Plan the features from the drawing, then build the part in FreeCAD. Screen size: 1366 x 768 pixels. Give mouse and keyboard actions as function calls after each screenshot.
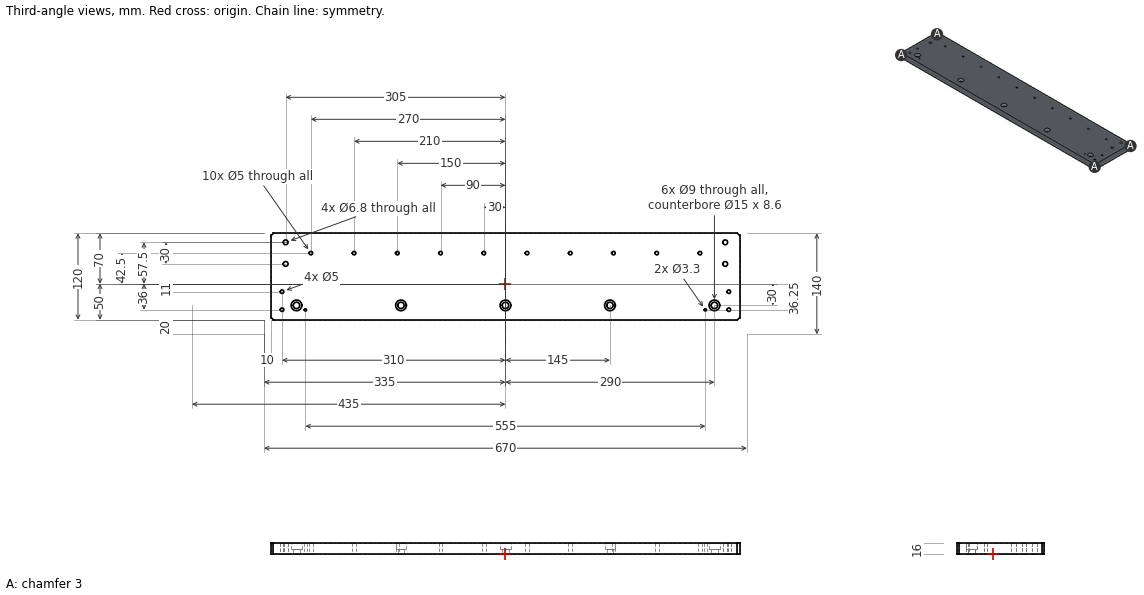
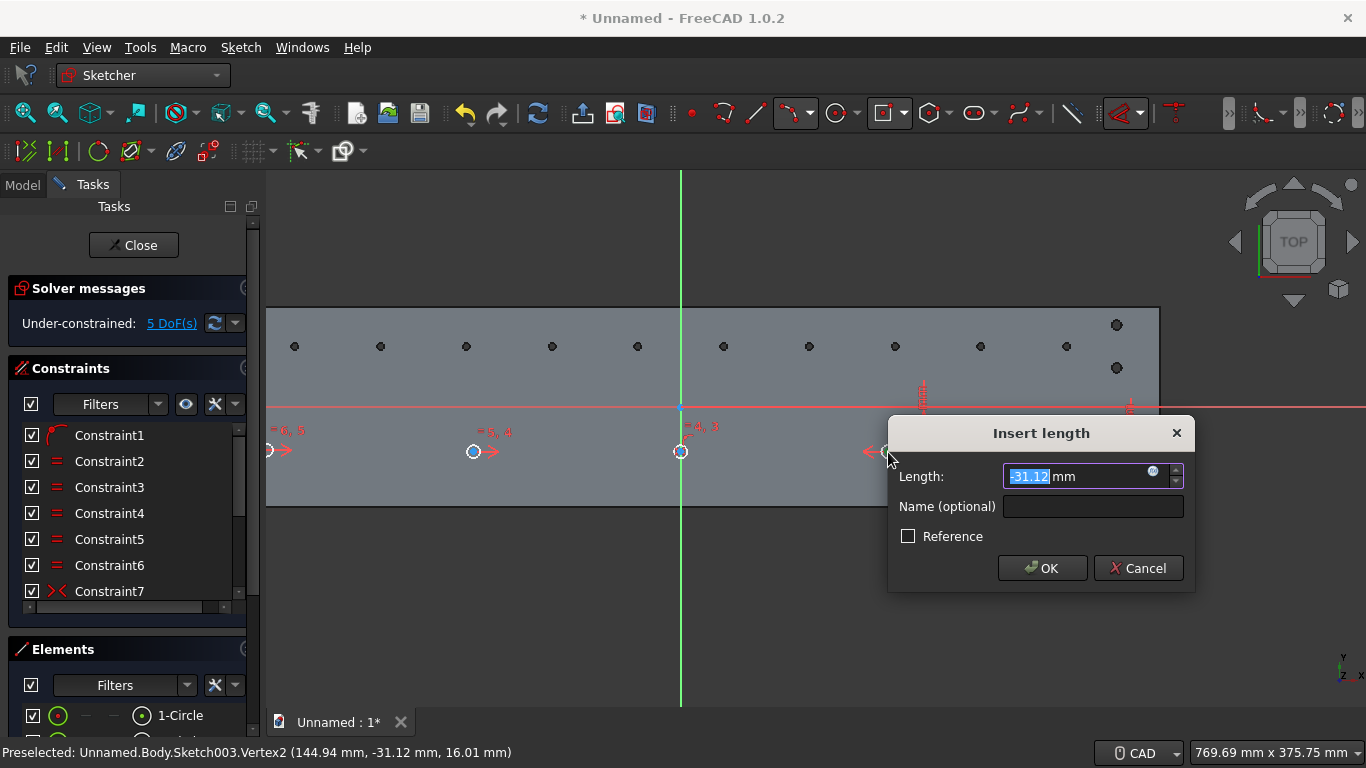
text(-30)
key(Return)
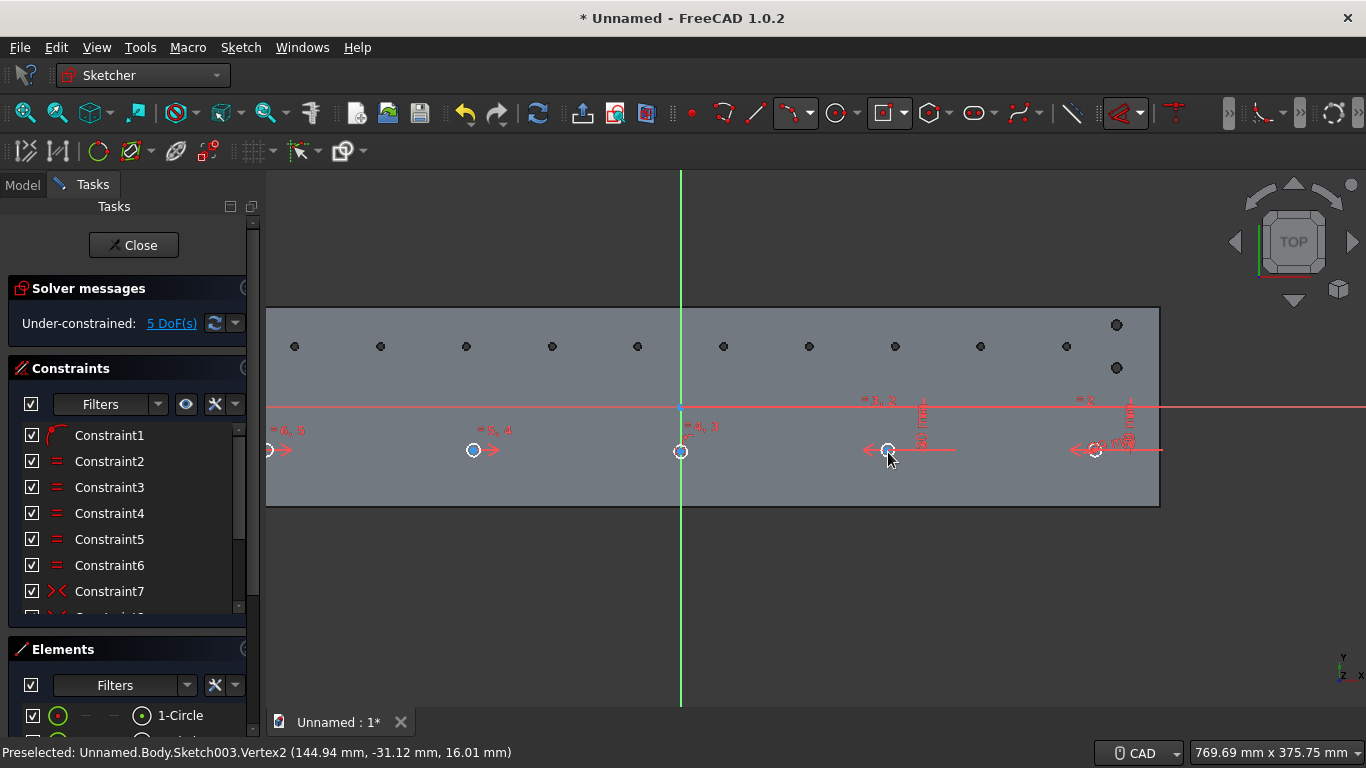
click(681, 452)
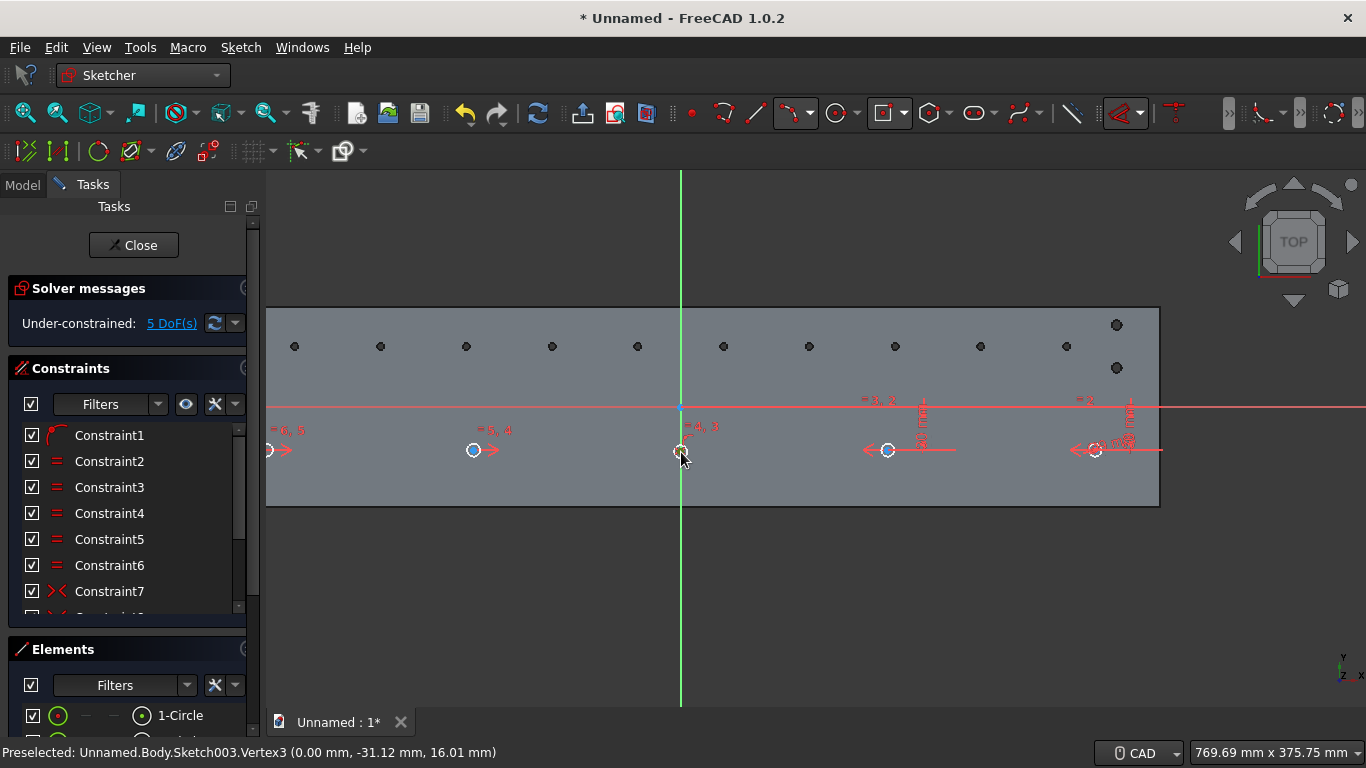
click(1142, 114)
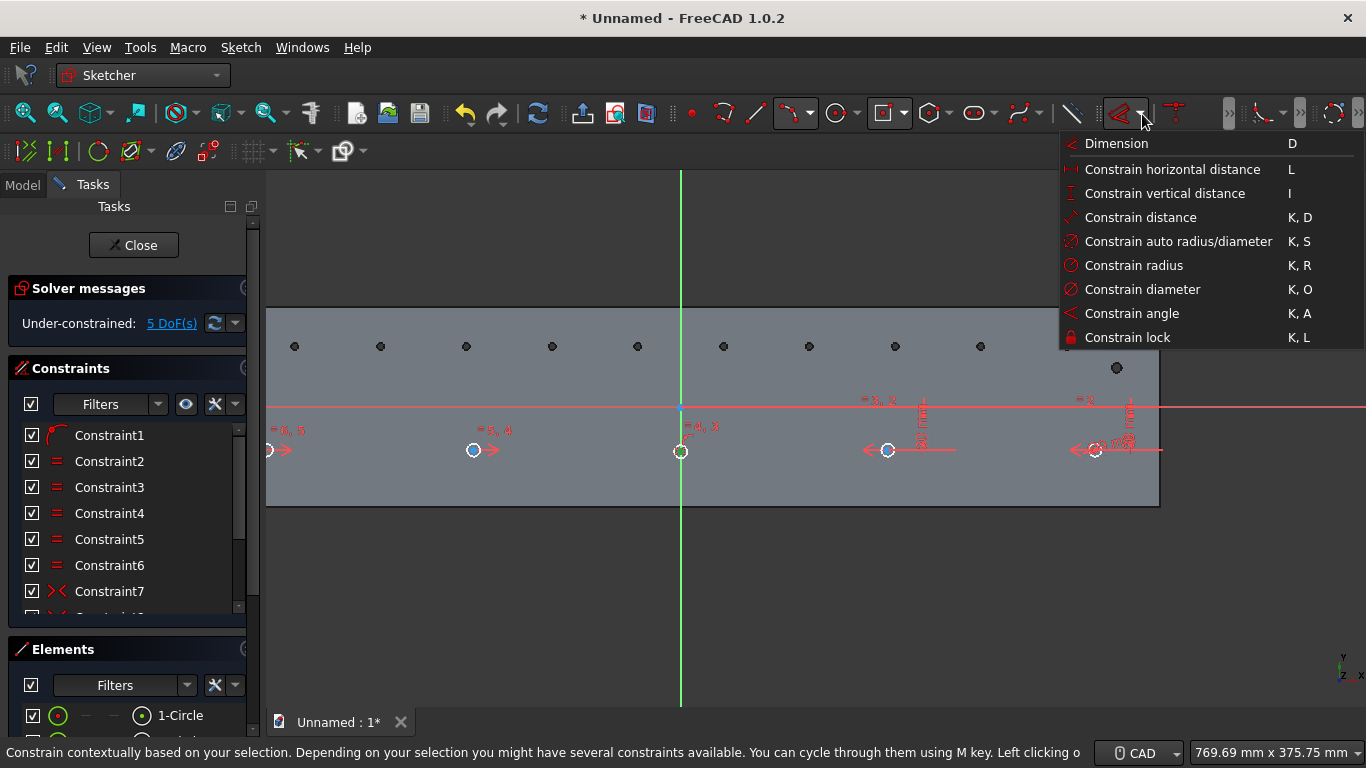
click(1212, 193)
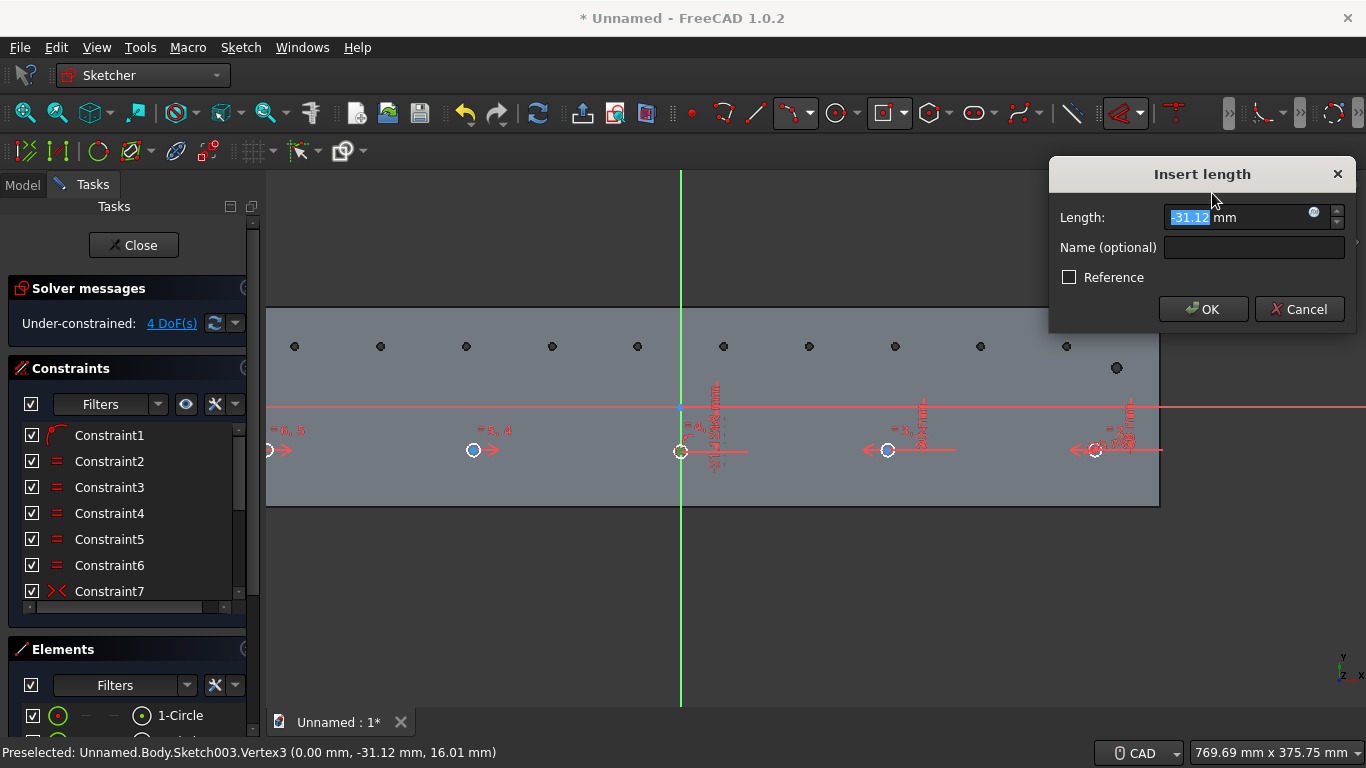
text(-30)
key(Return)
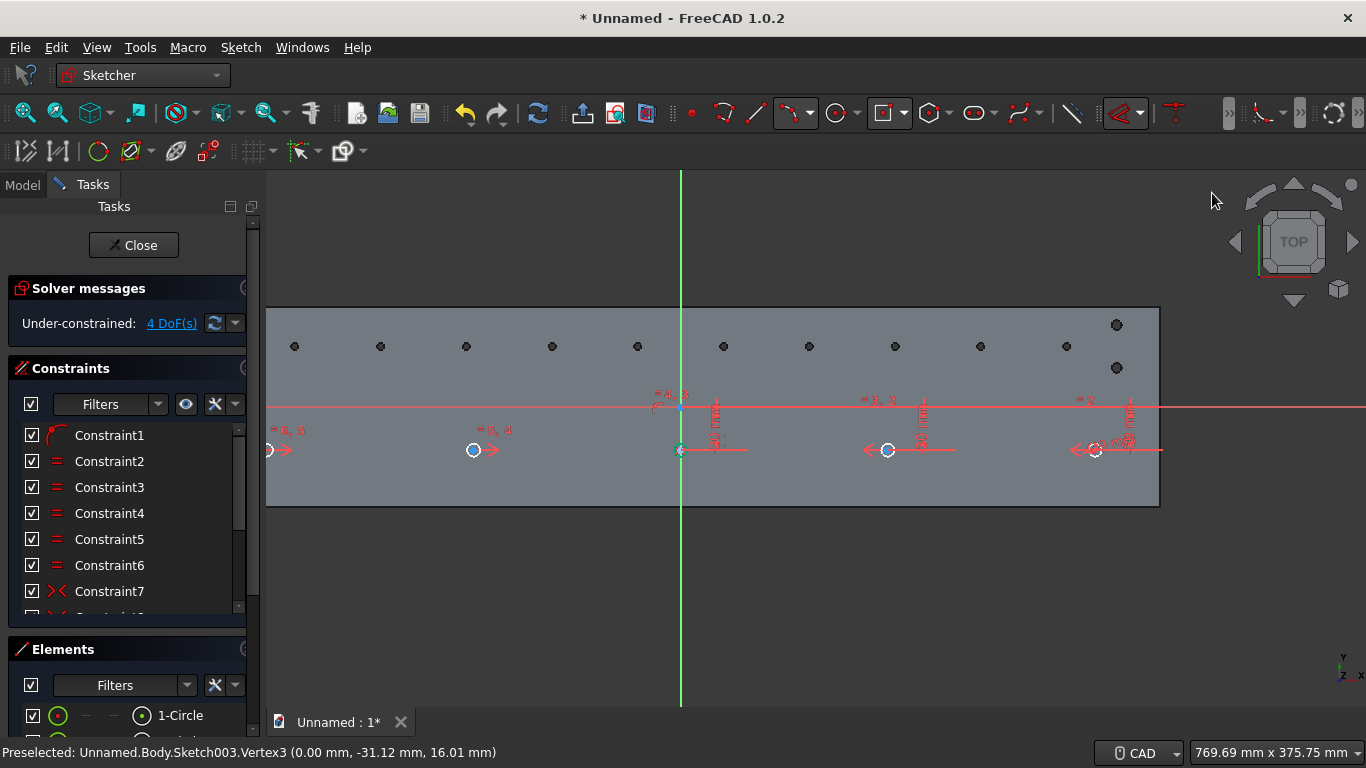
scroll(1094, 452, down, 2)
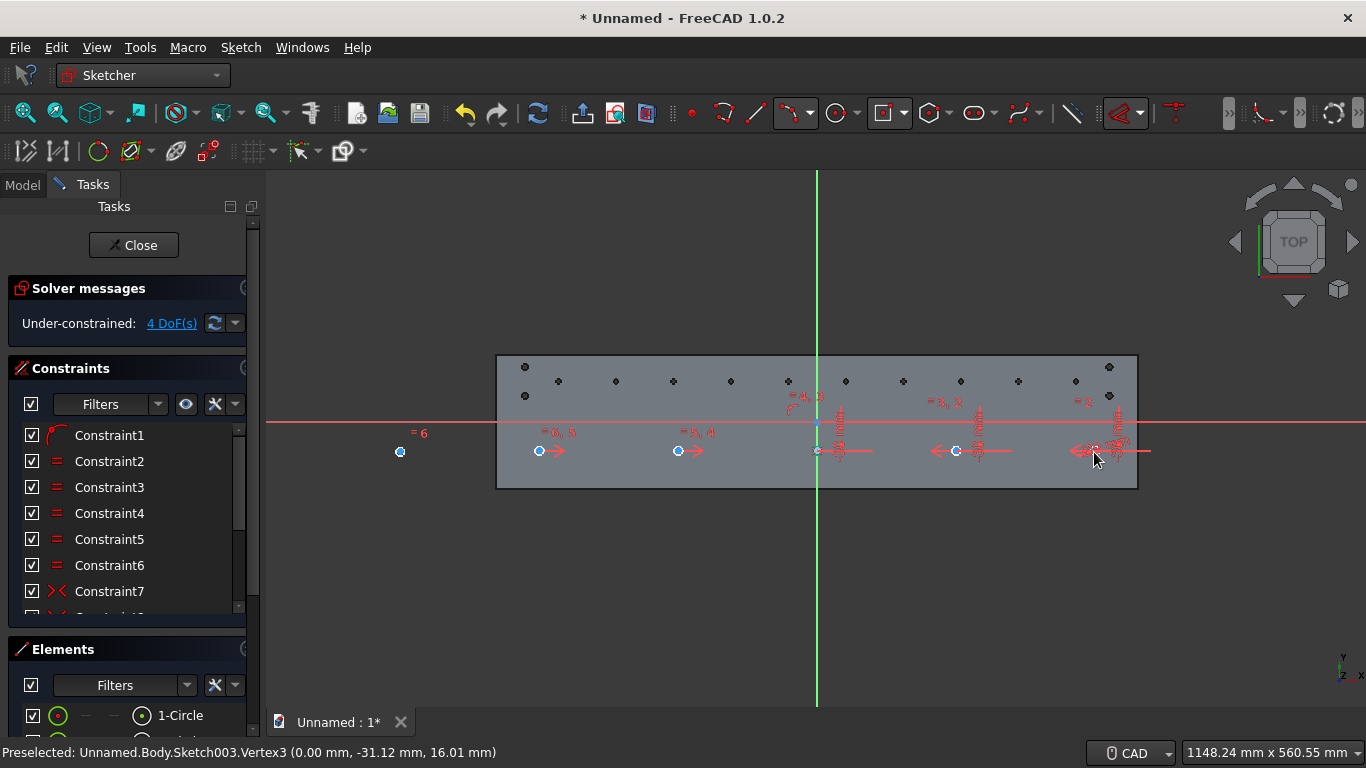
scroll(400, 452, up, 2)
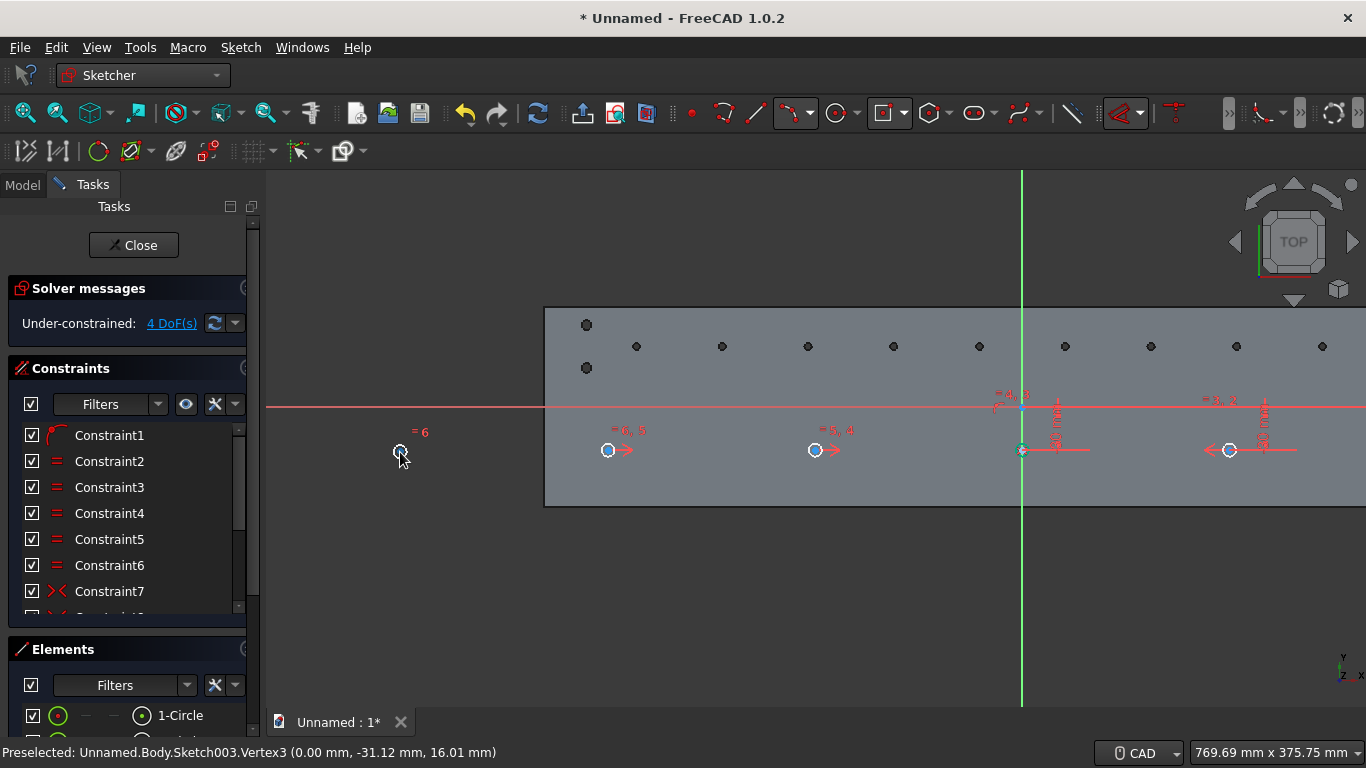
click(400, 452)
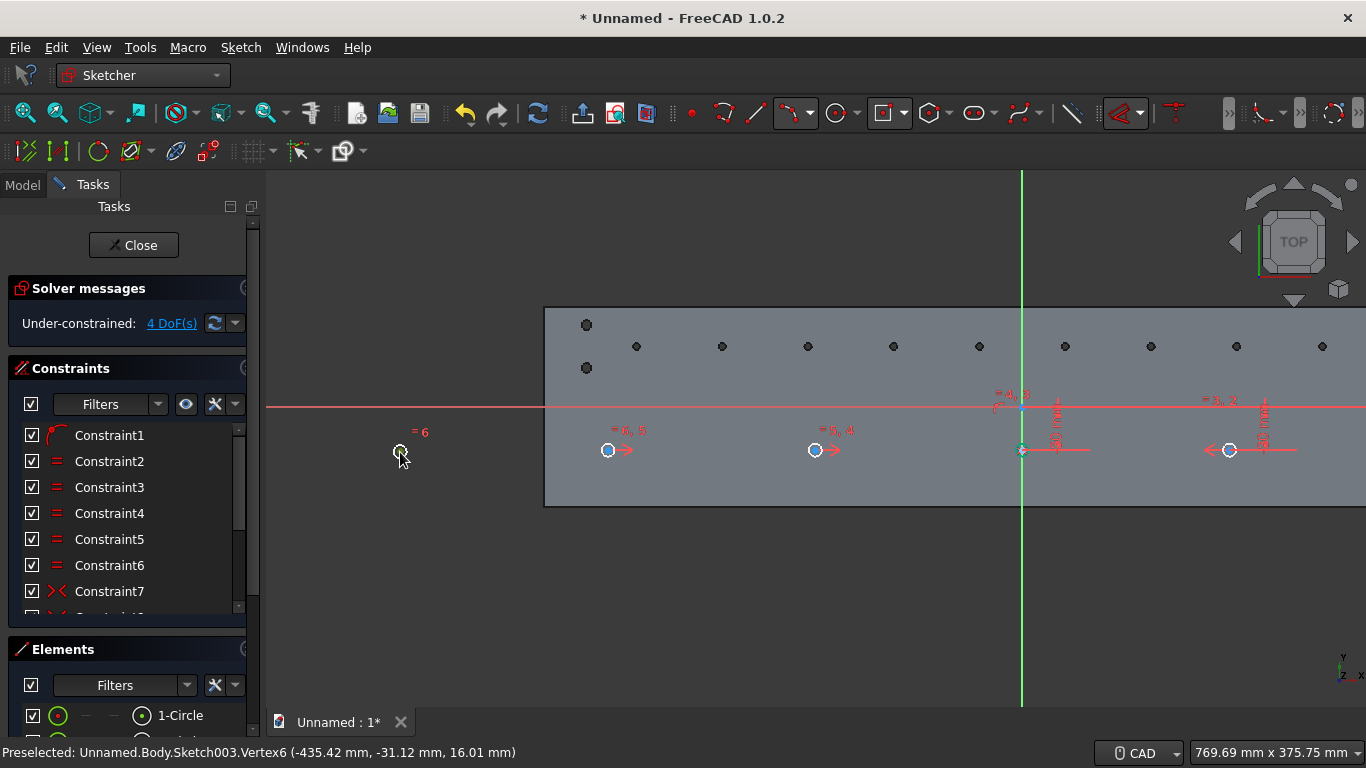
click(1142, 114)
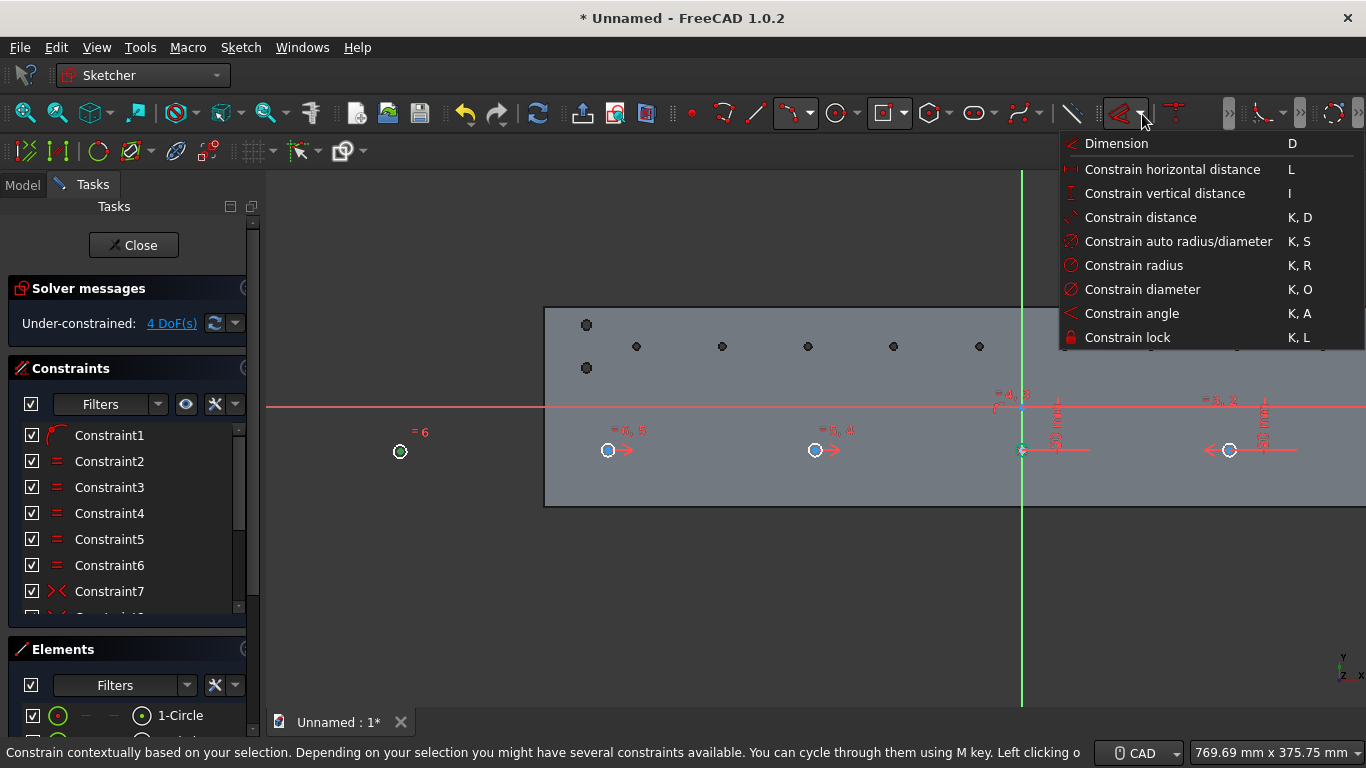
click(1212, 193)